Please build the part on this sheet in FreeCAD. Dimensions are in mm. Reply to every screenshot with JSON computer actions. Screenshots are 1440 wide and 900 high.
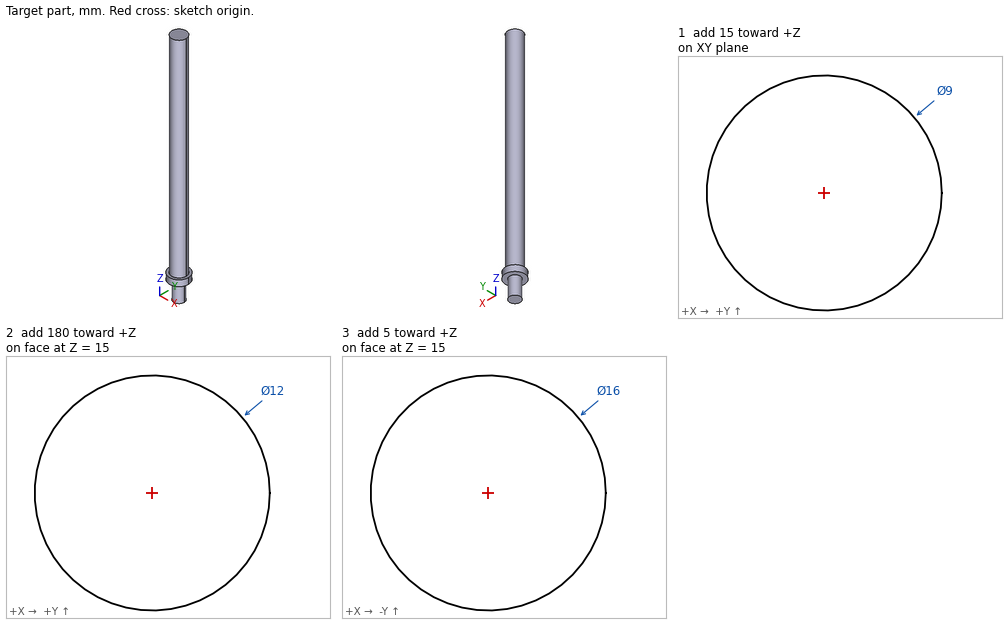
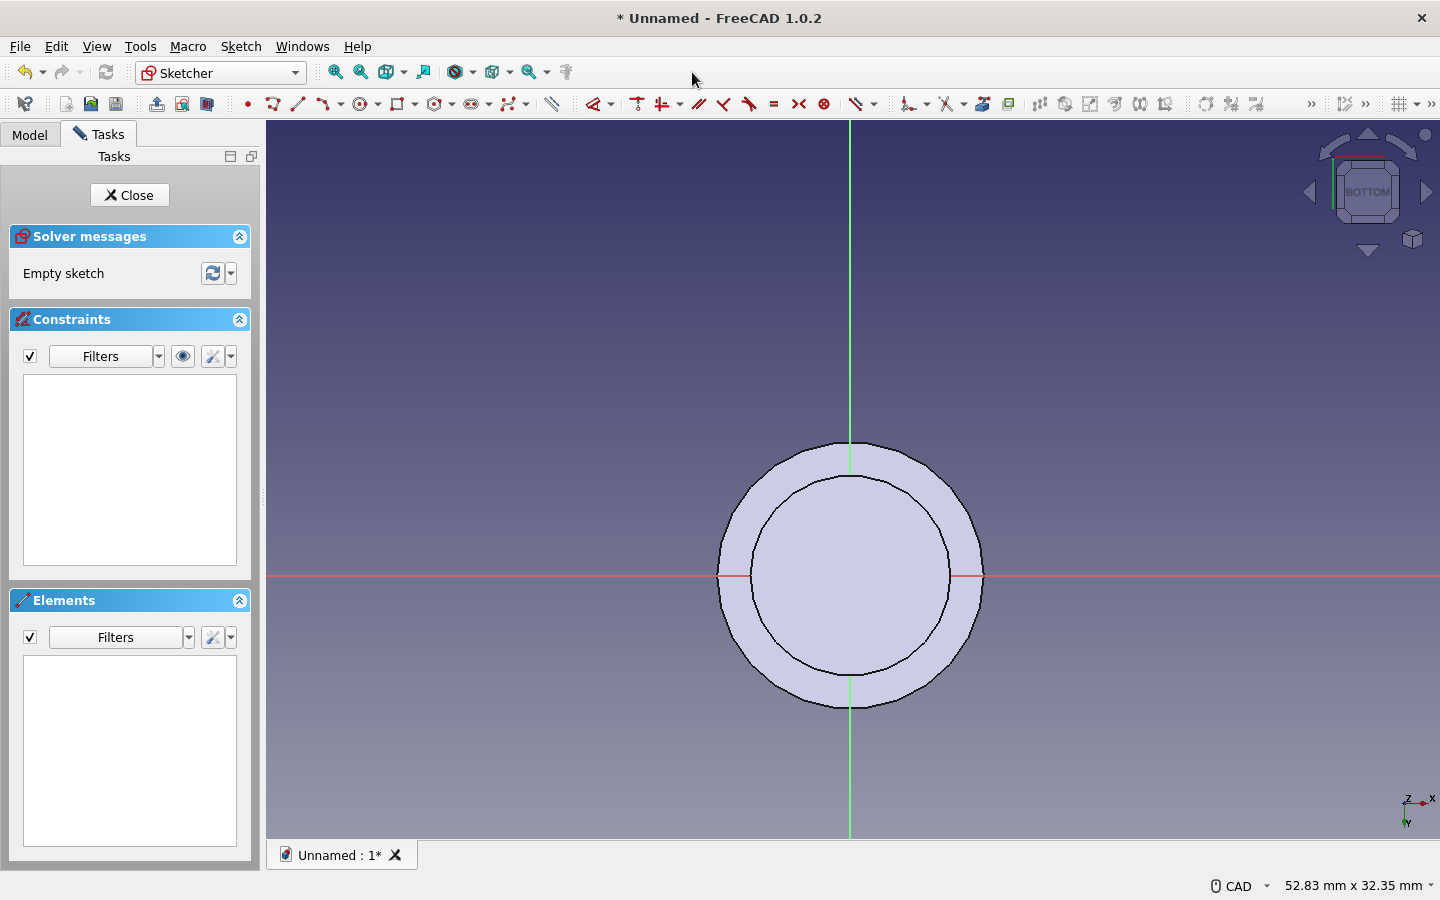
{"action": "key", "text": "q s"}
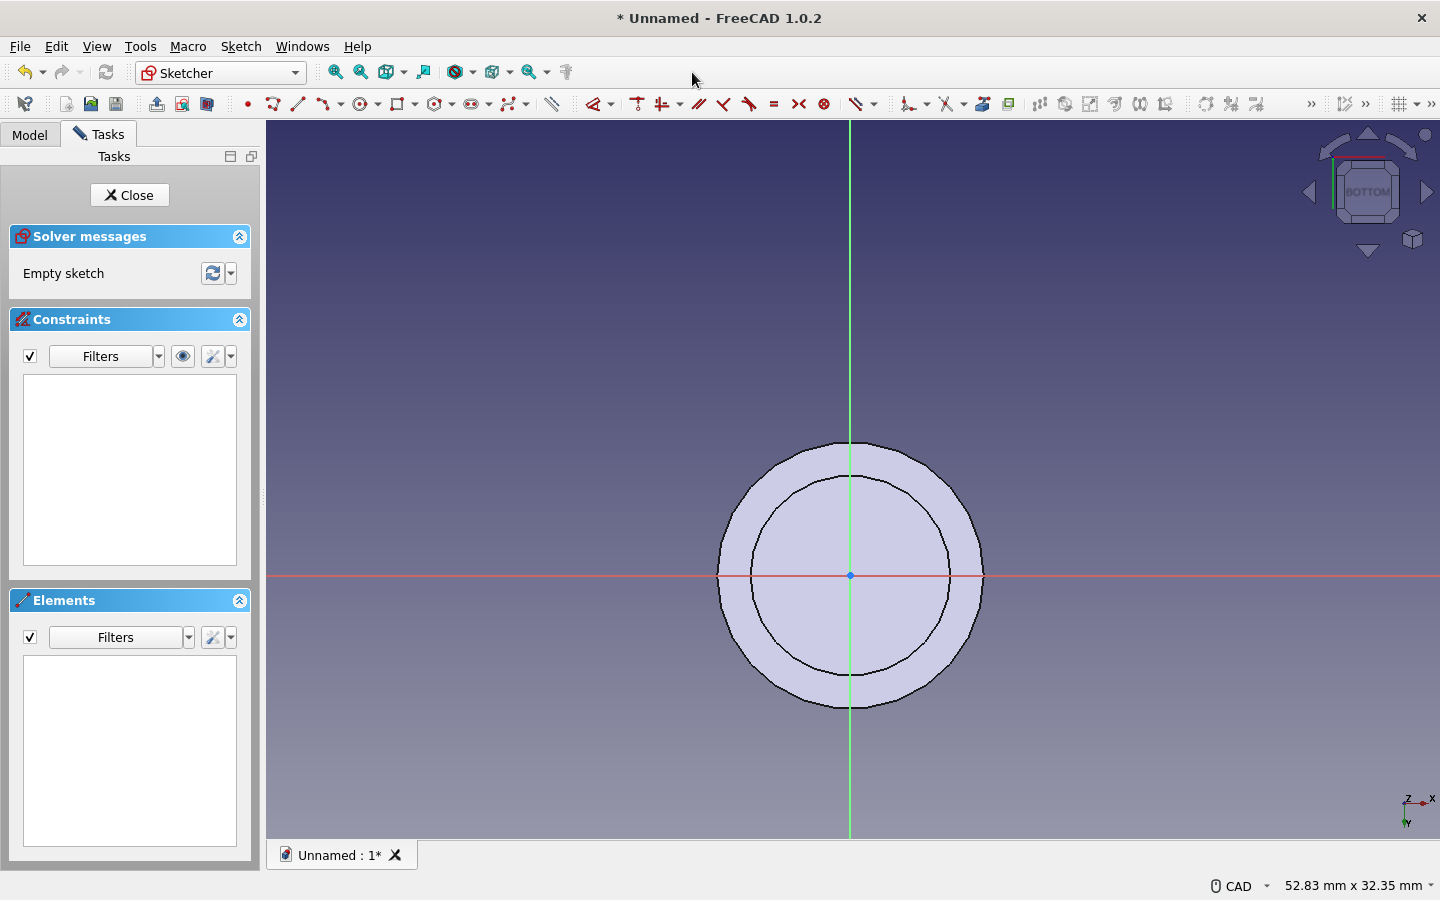
{"action": "key", "text": "g c"}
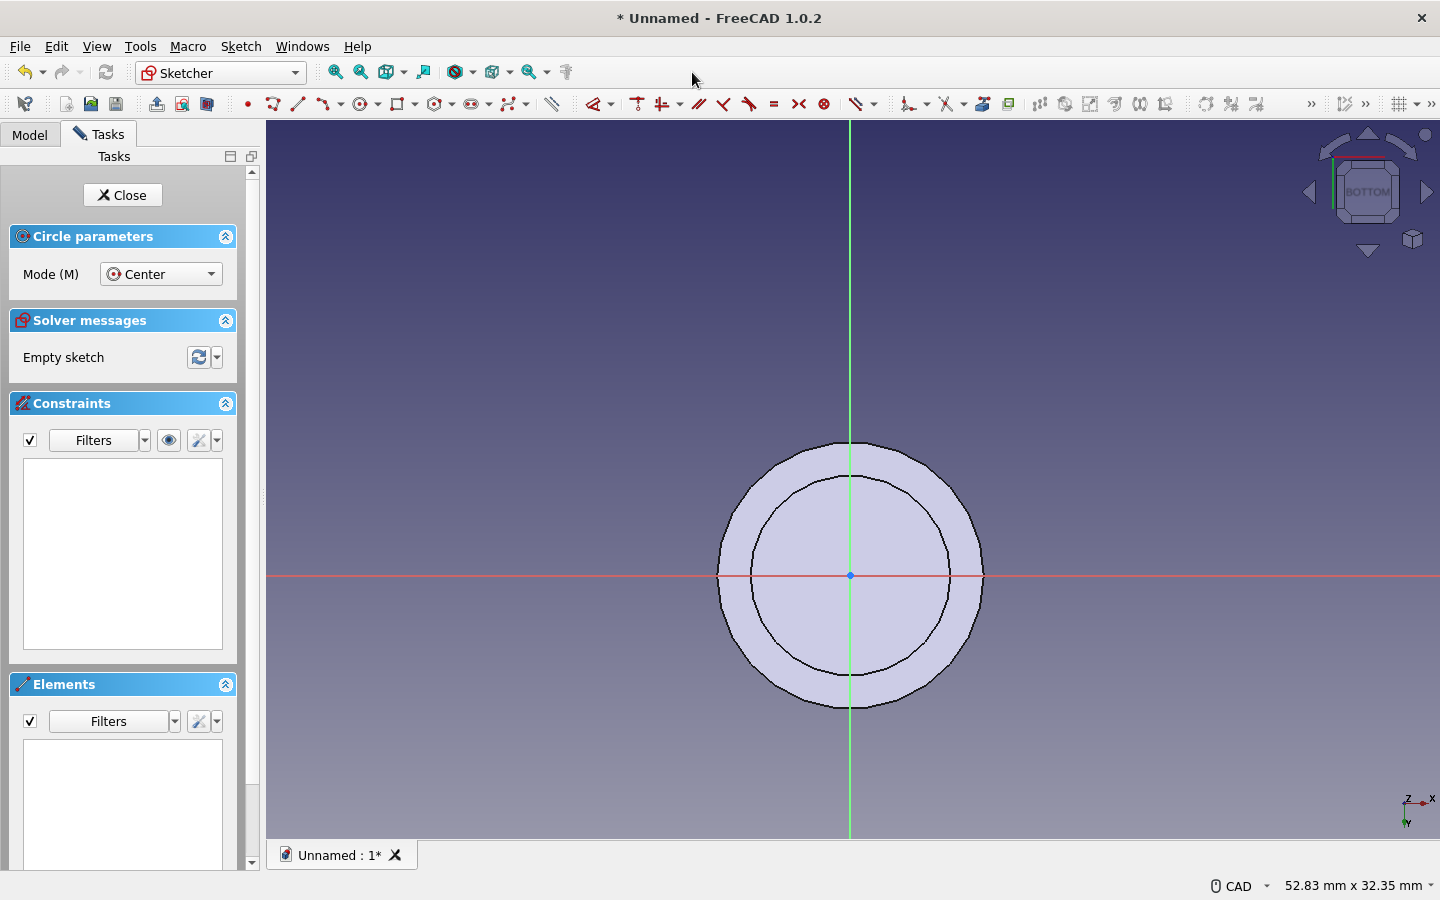
{"action": "left_click", "coordinate": [850, 576]}
{"action": "left_click", "coordinate": [976, 450]}
{"action": "key", "text": "Escape"}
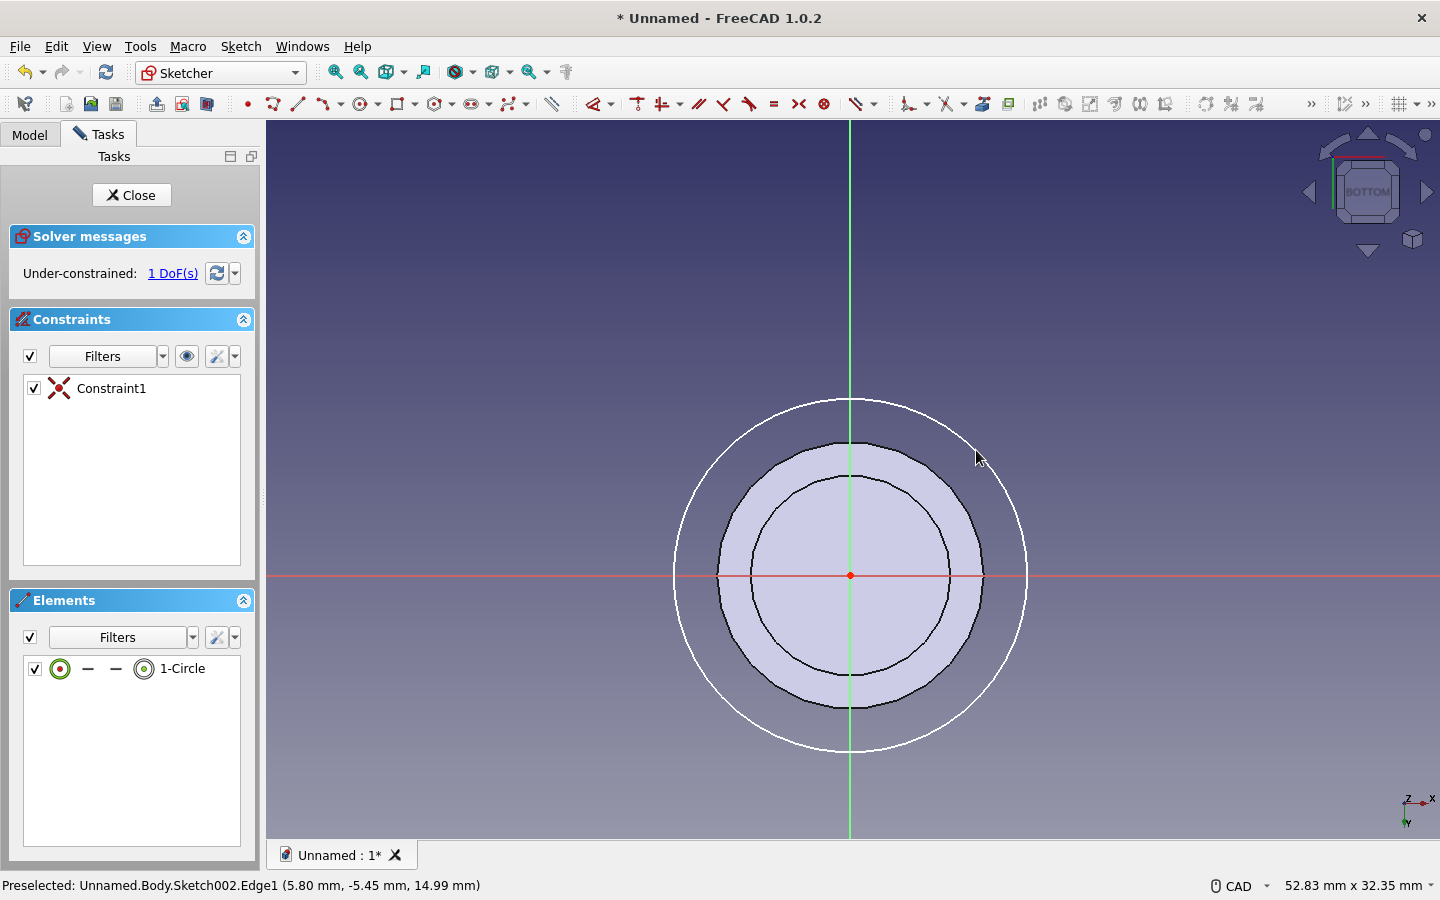
{"action": "key", "text": "d"}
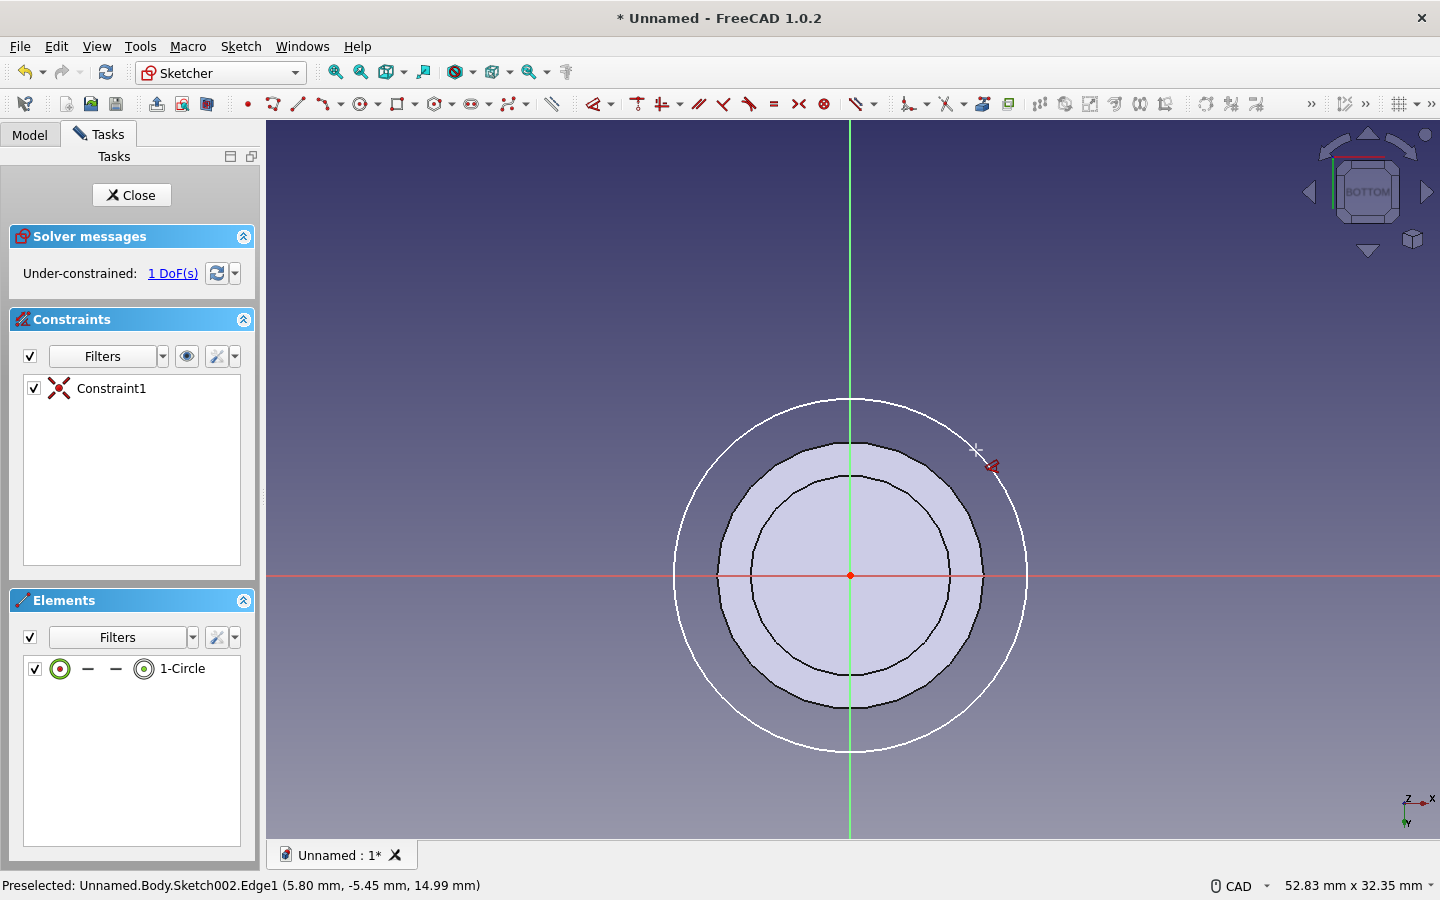
{"action": "left_click", "coordinate": [975, 450]}
{"action": "left_click", "coordinate": [998, 427]}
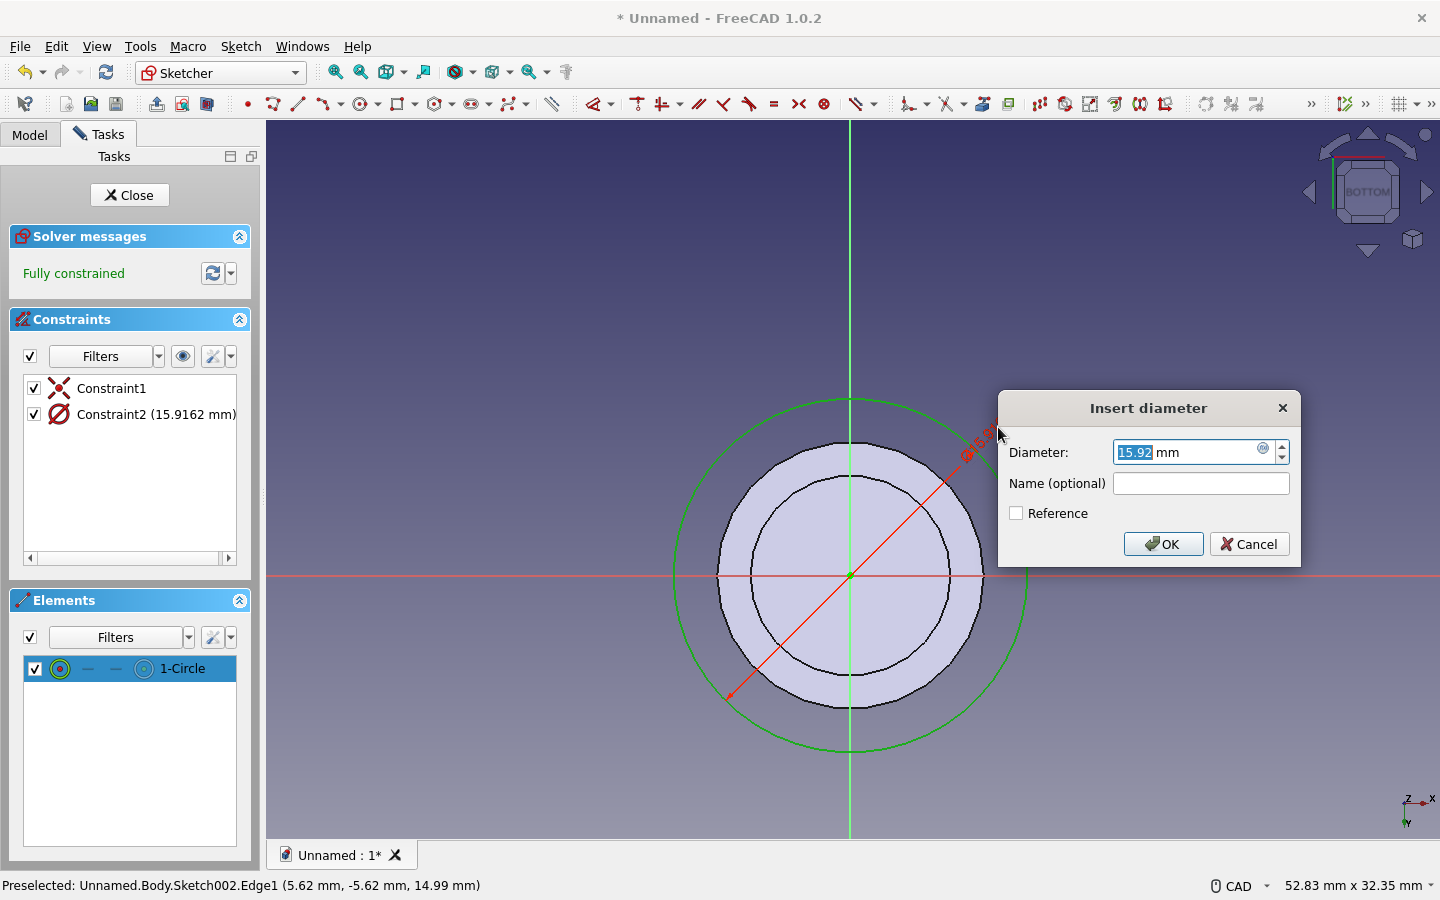
{"action": "type", "text": "16"}
{"action": "key", "text": "Return"}
{"action": "key", "text": "Escape"}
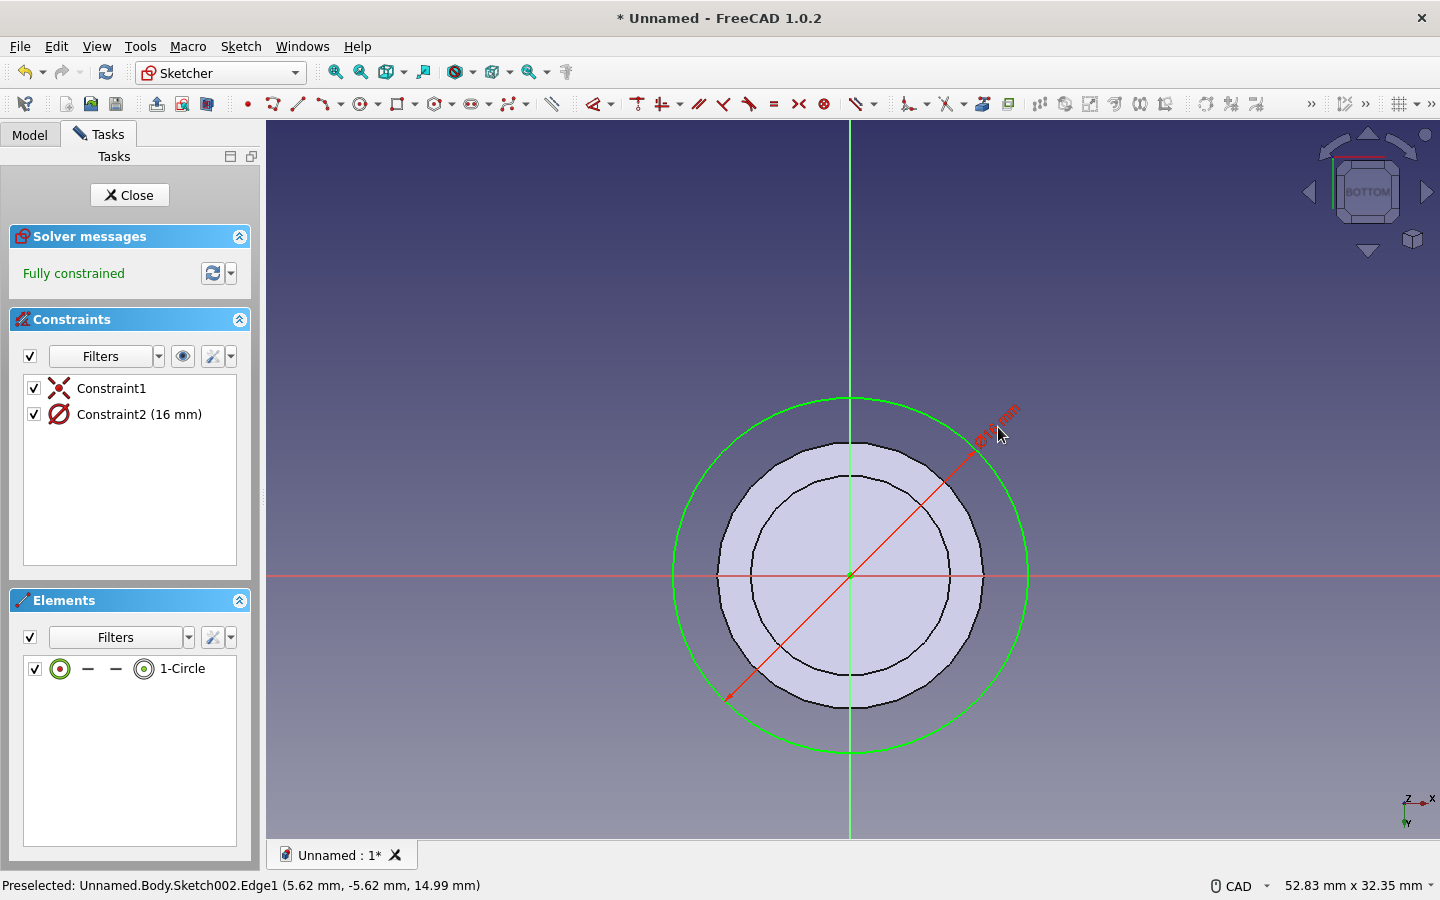
{"action": "left_click", "coordinate": [130, 195]}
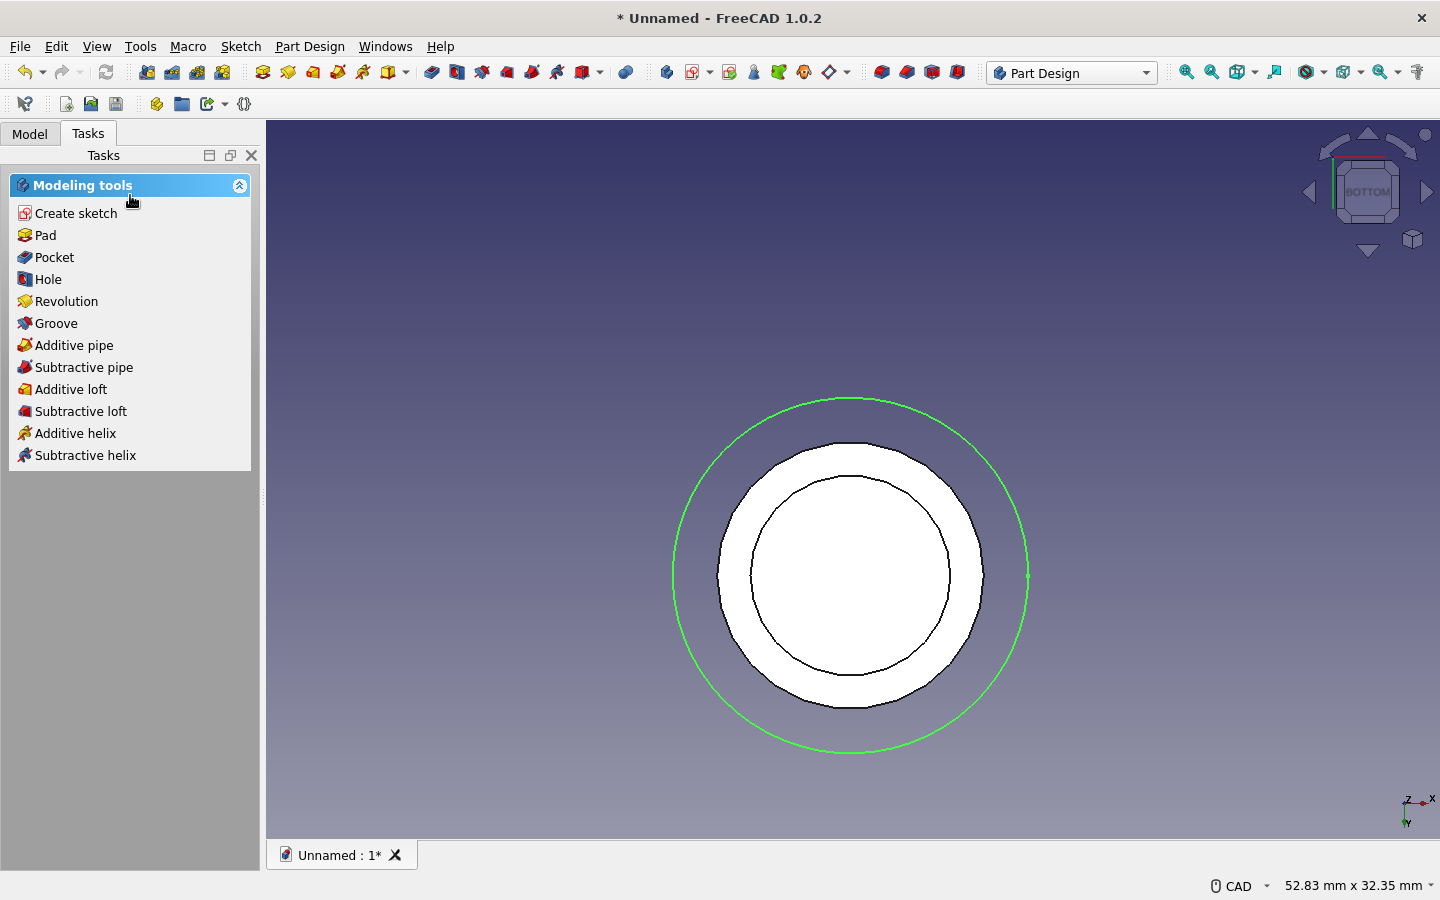
{"action": "left_click", "coordinate": [263, 72]}